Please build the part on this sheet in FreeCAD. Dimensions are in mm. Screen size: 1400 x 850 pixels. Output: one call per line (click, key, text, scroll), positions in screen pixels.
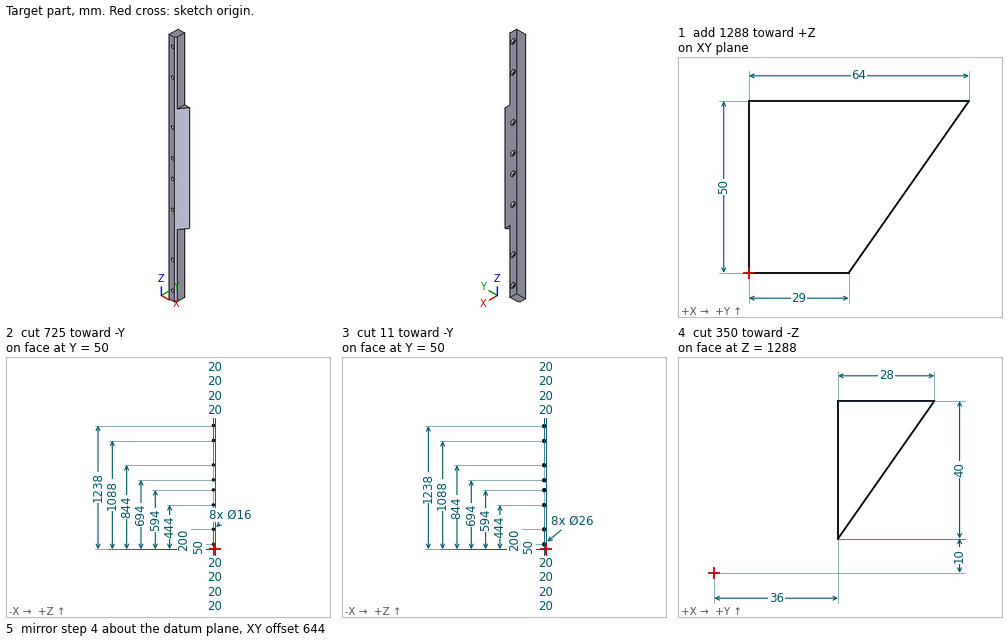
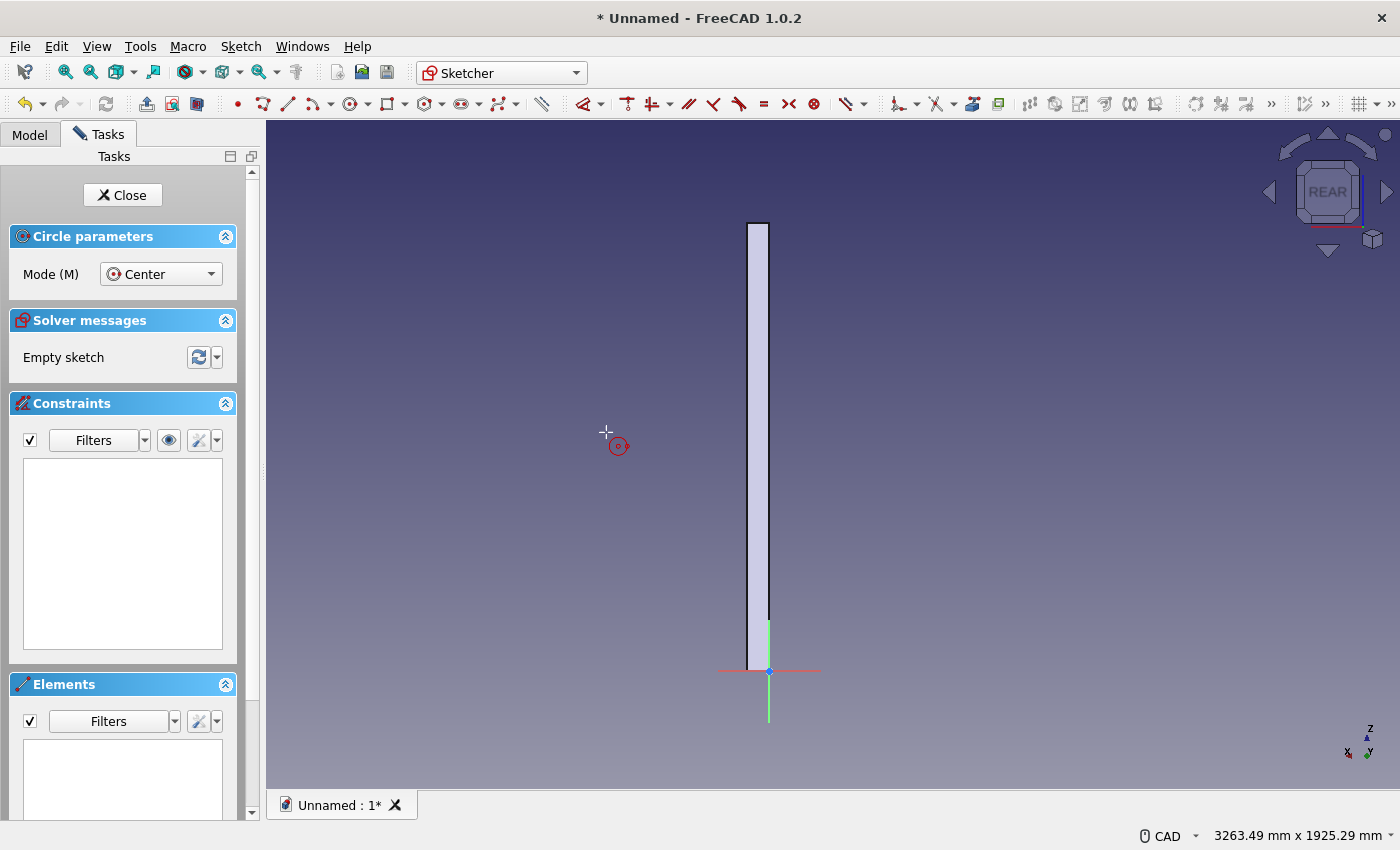
scroll(762, 654, up, 11)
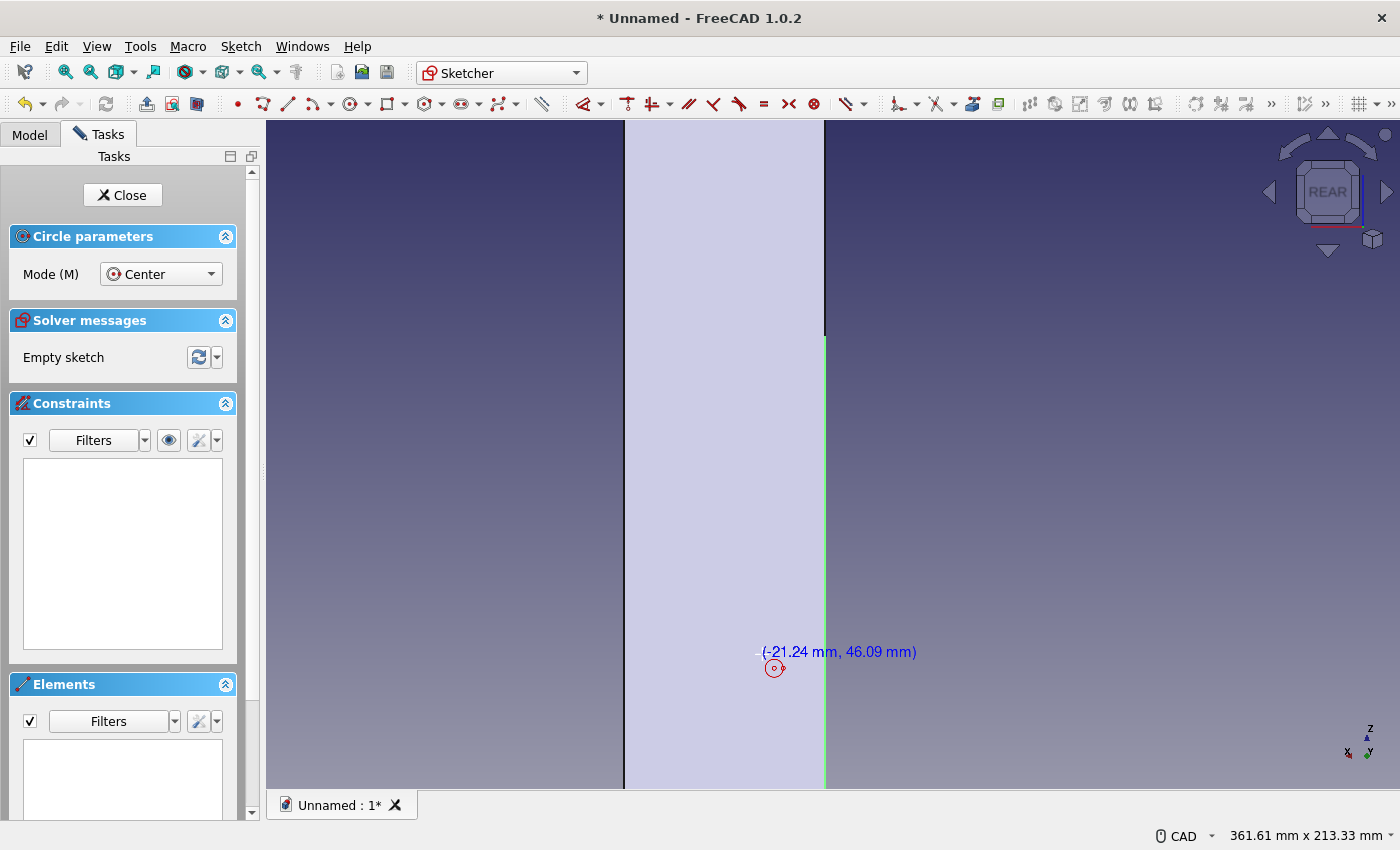
scroll(762, 655, down, 11)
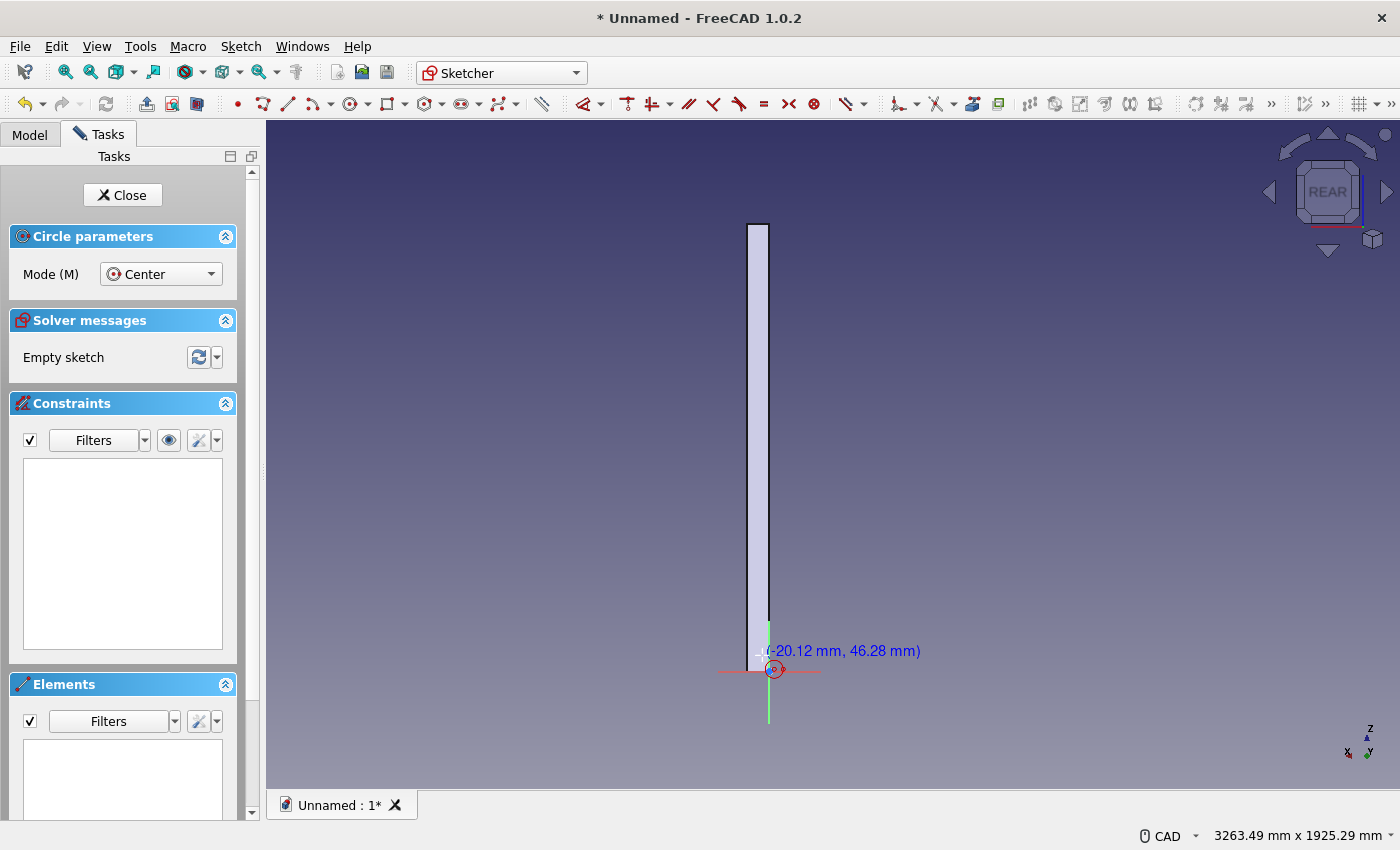
scroll(762, 655, up, 5)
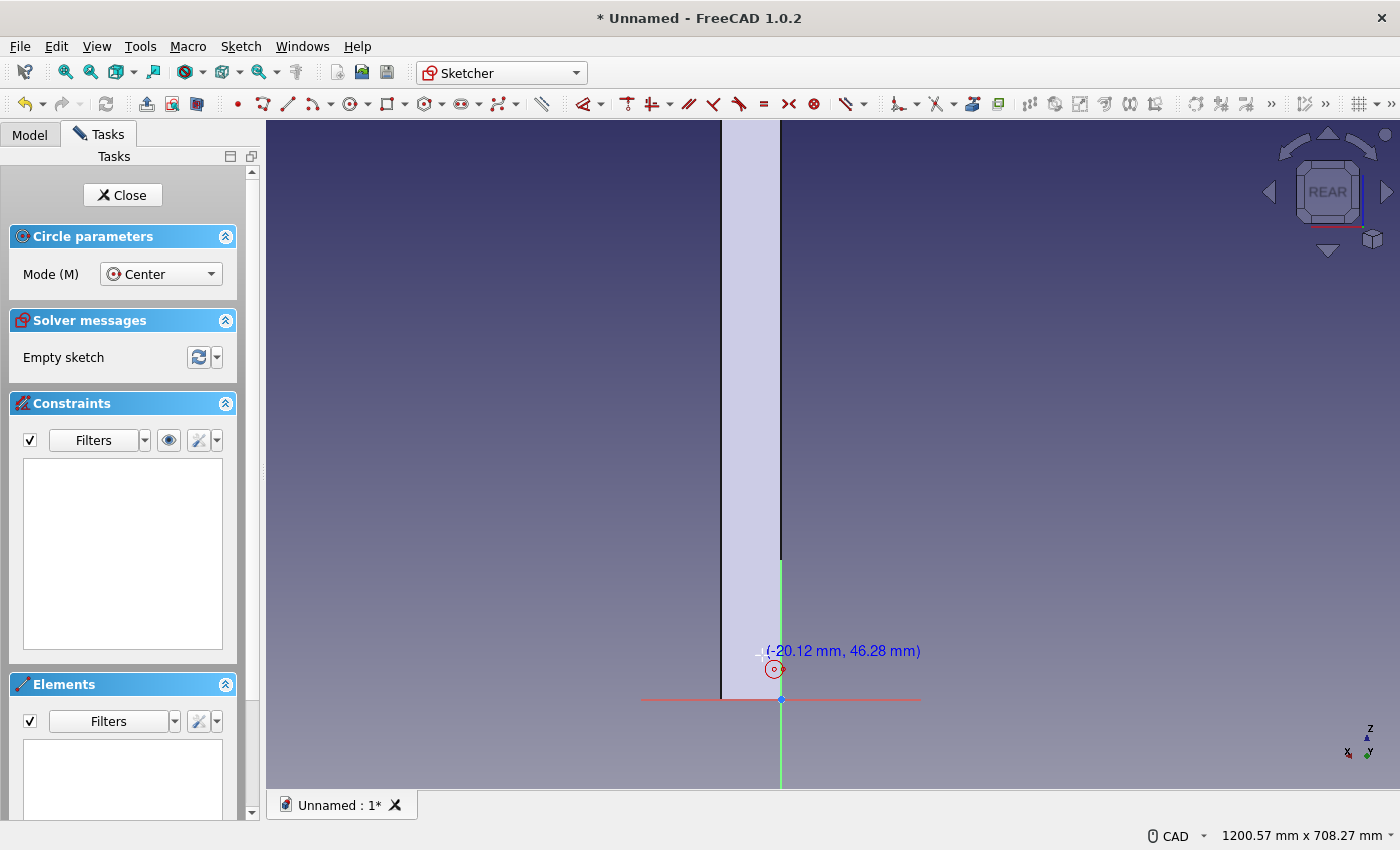
click(762, 652)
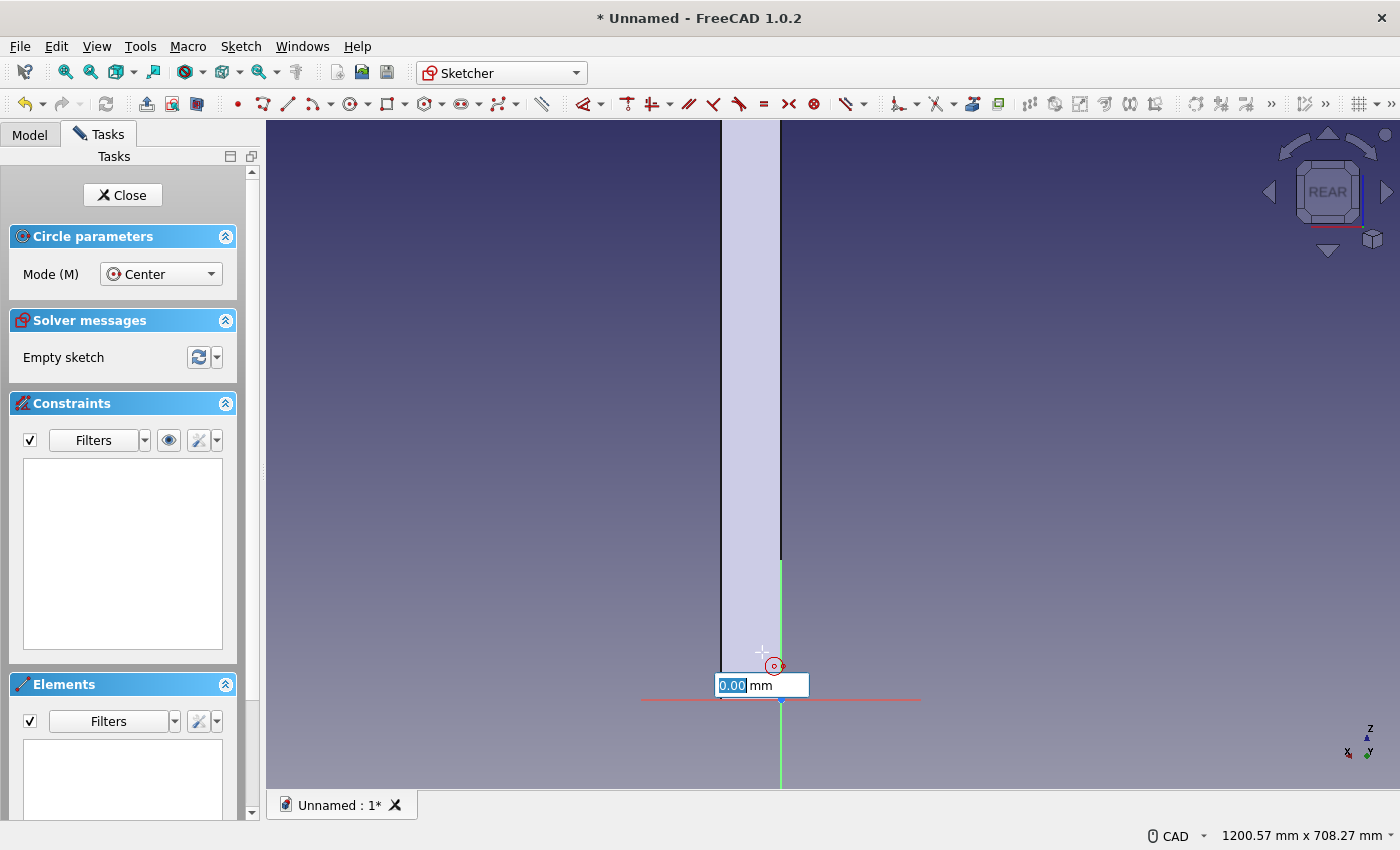
scroll(757, 647, up, 4)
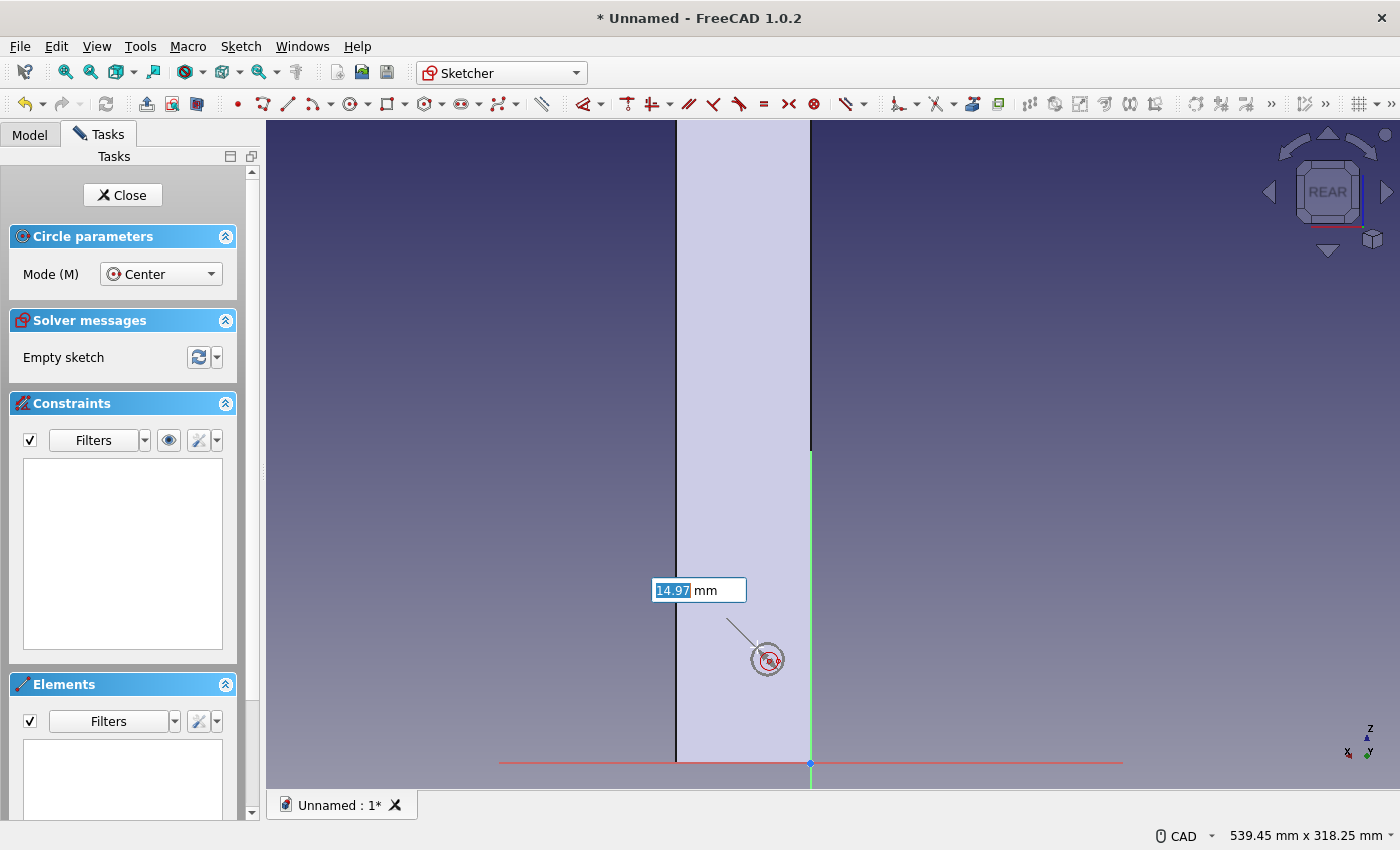
click(757, 646)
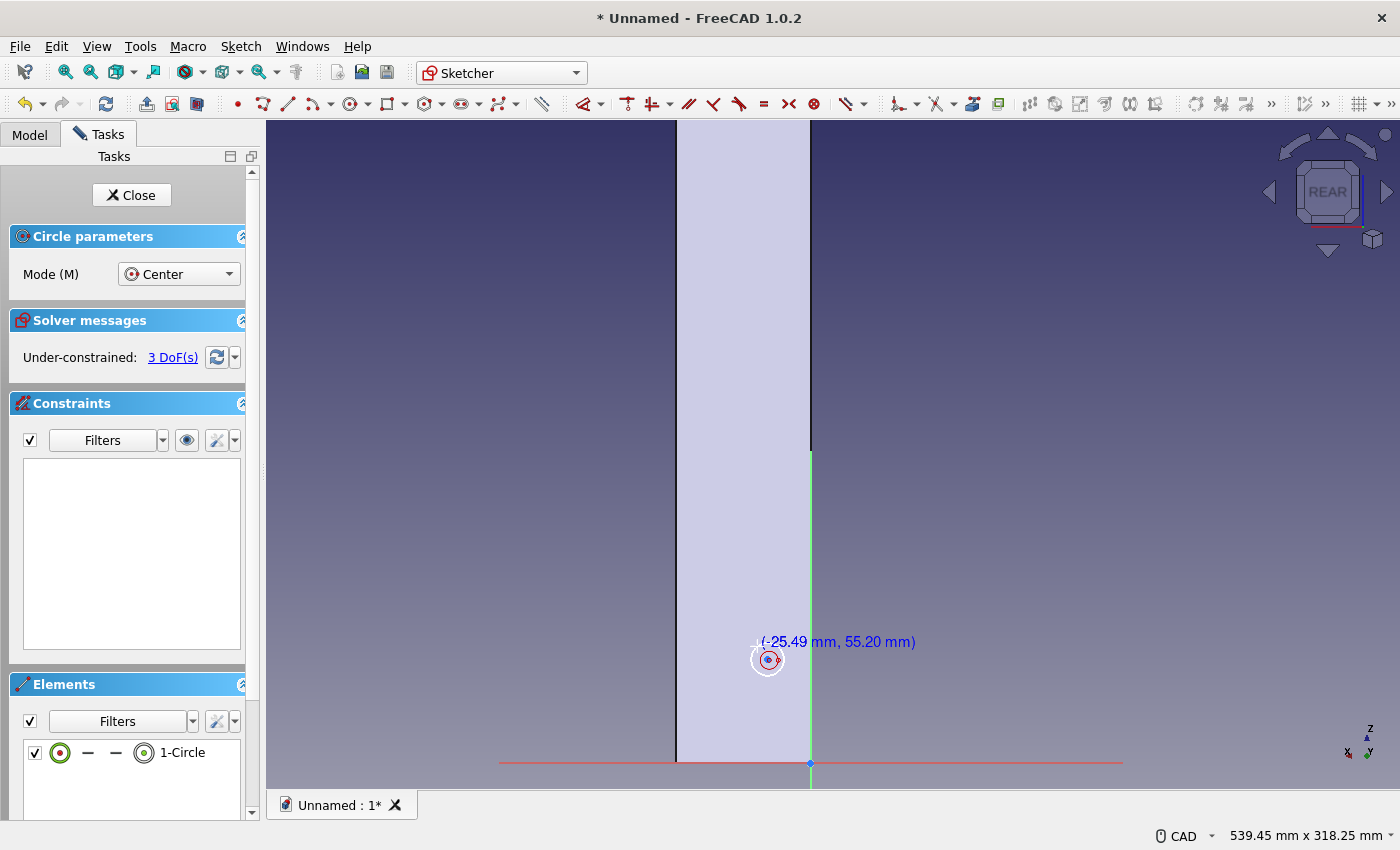
scroll(769, 343, up, 2)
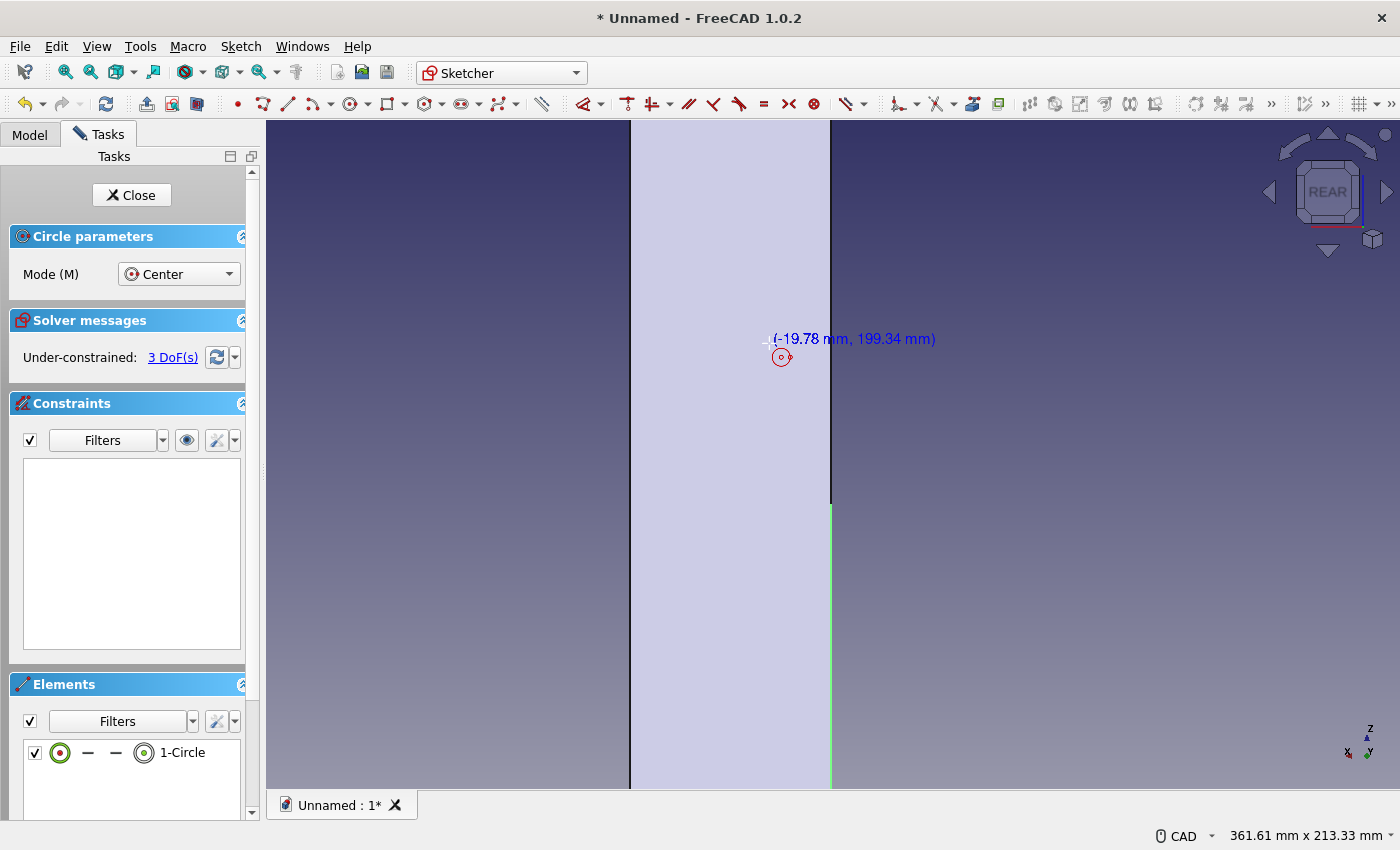
scroll(762, 634, down, 11)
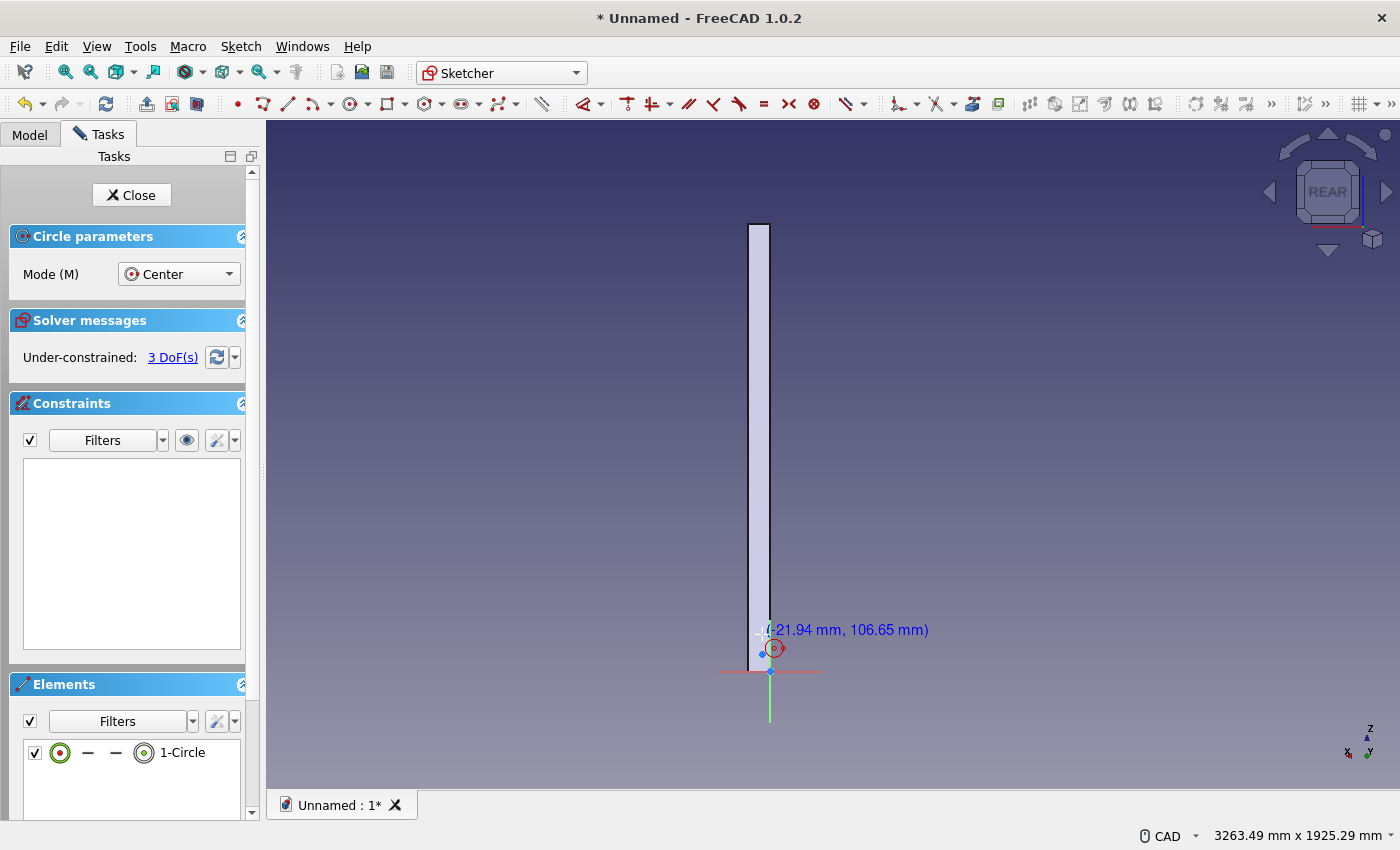
scroll(763, 602, up, 5)